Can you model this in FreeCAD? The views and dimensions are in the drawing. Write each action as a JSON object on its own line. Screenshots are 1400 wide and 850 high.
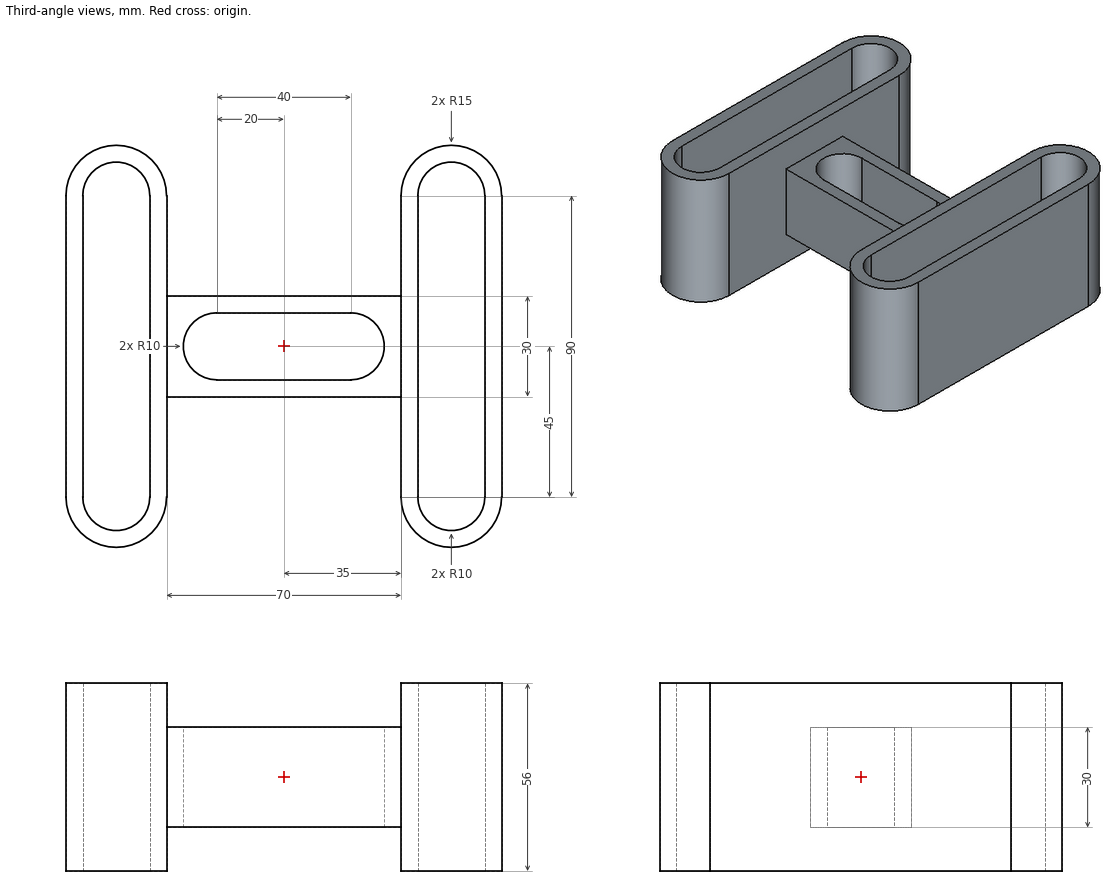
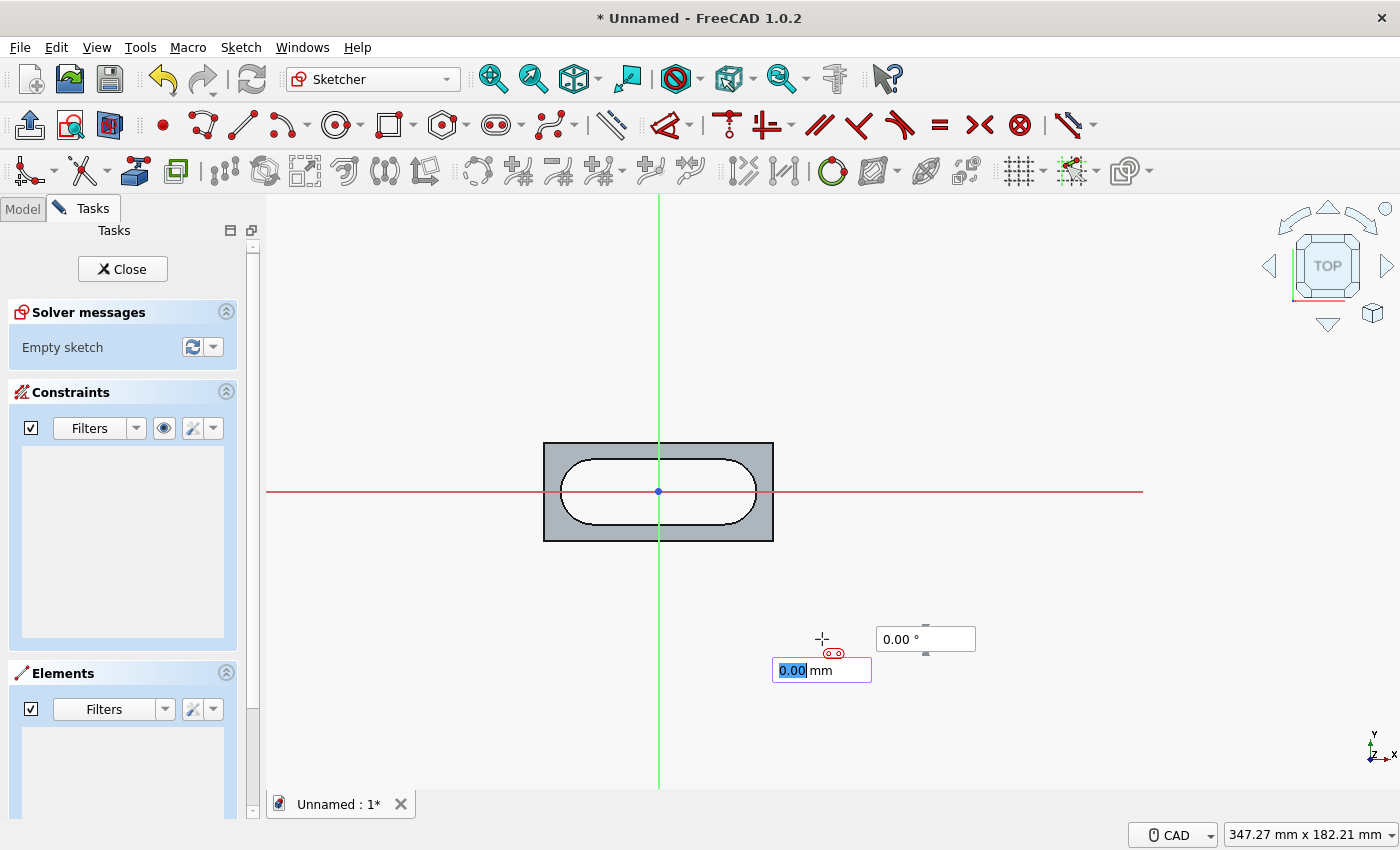
{"action": "left_click", "coordinate": [822, 345]}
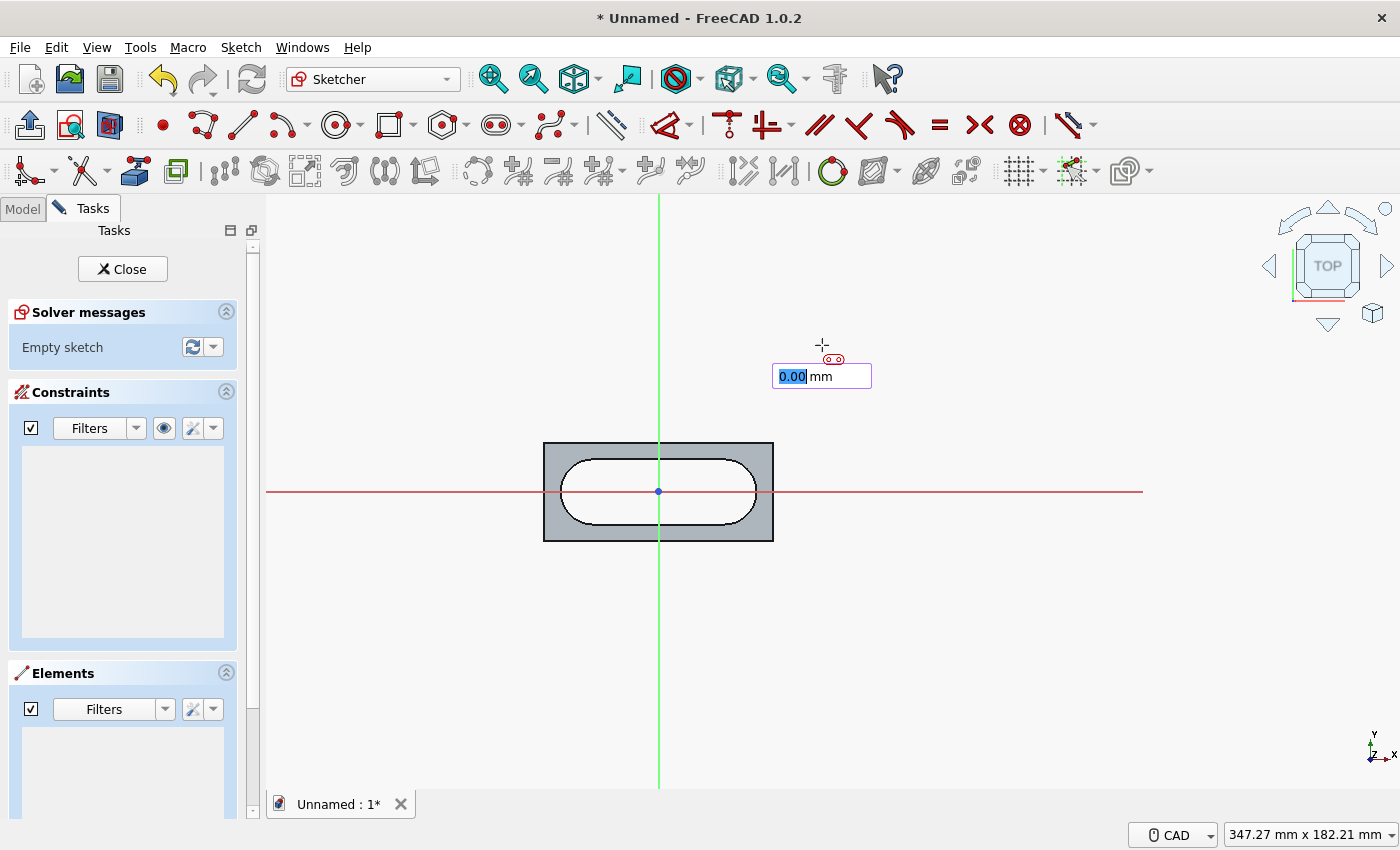
{"action": "left_click", "coordinate": [773, 448]}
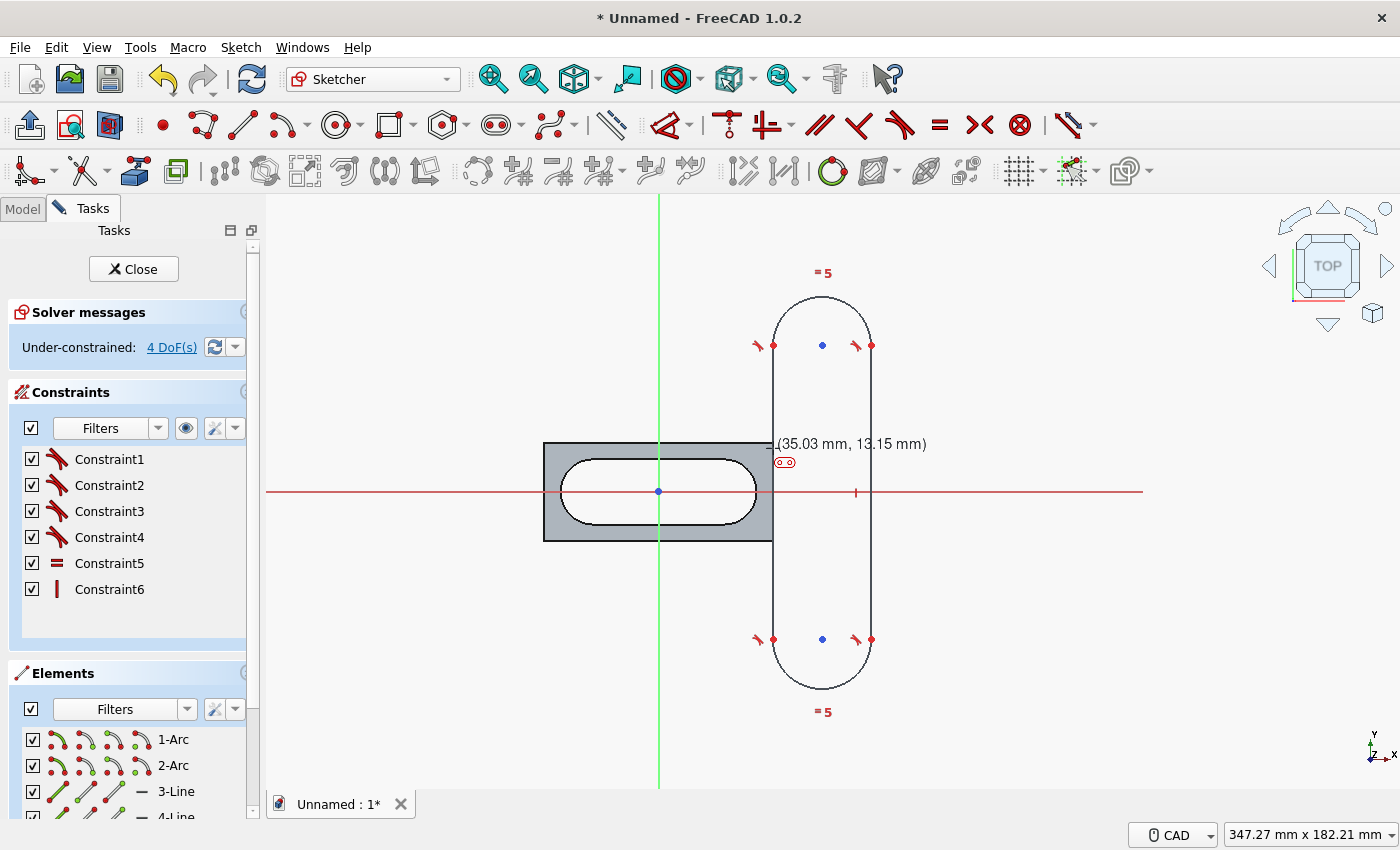
{"action": "left_click", "coordinate": [822, 640]}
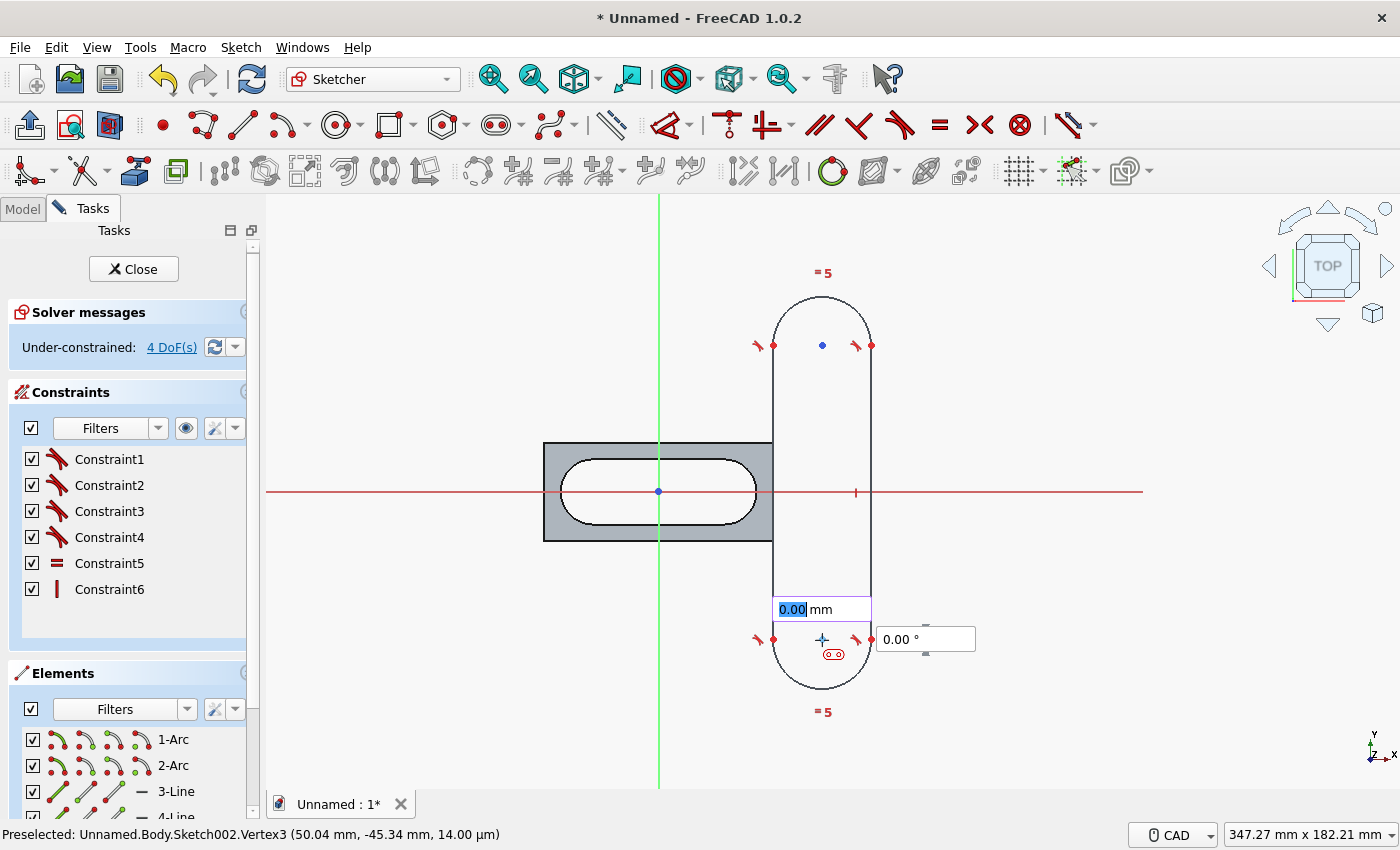
{"action": "left_click", "coordinate": [822, 346]}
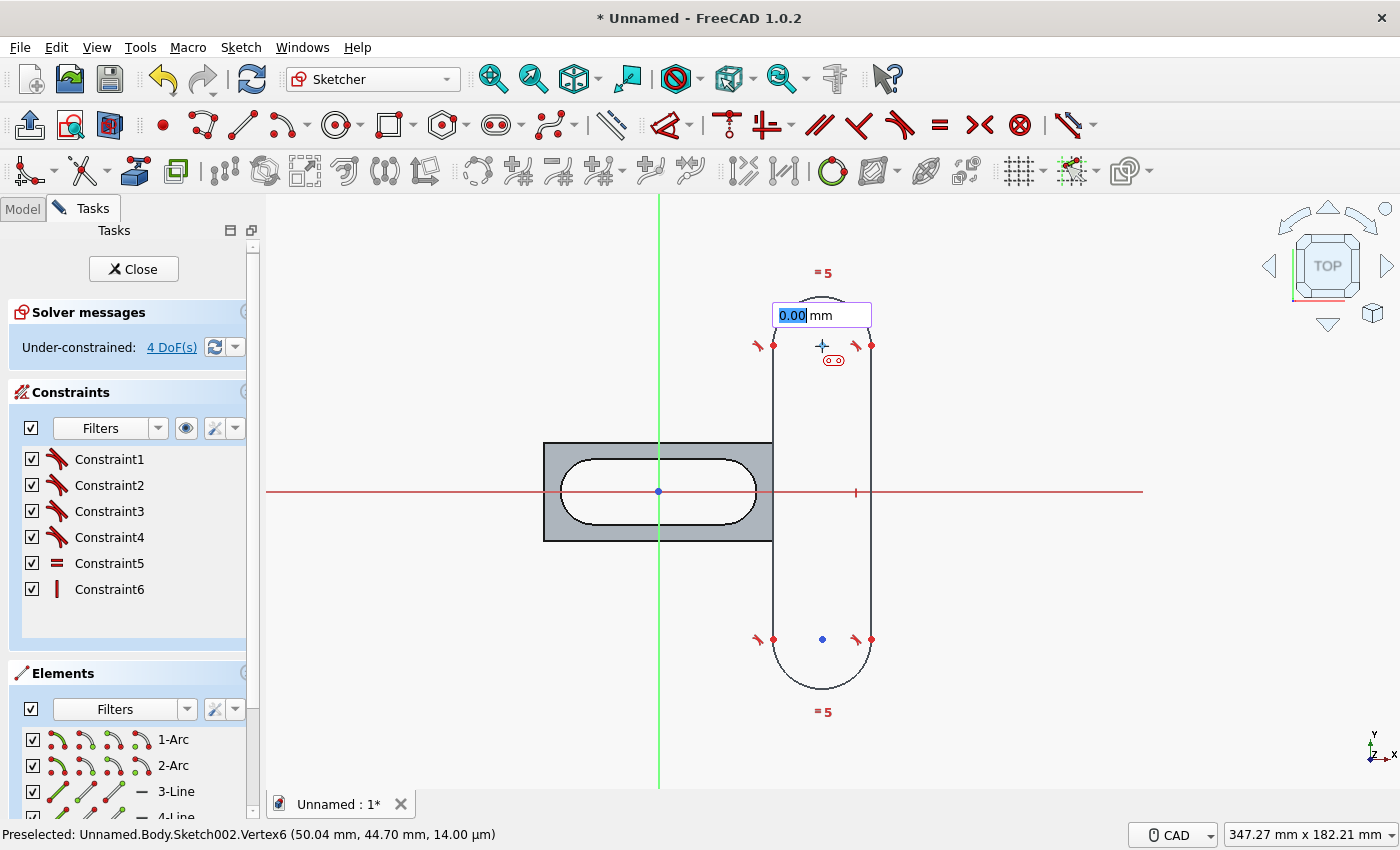
{"action": "left_click", "coordinate": [855, 448]}
{"action": "key", "text": "Escape"}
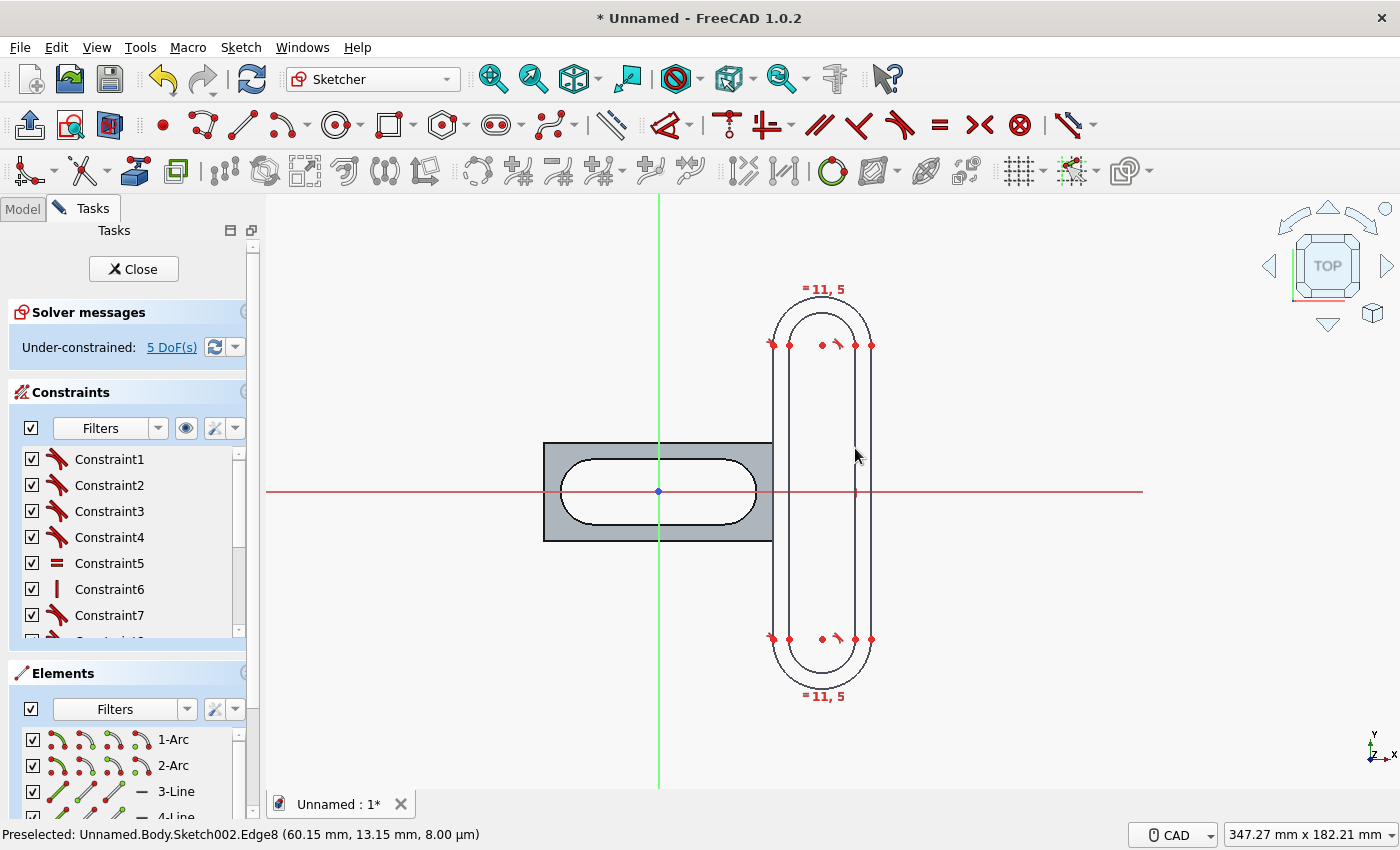
{"action": "left_click", "coordinate": [793, 680]}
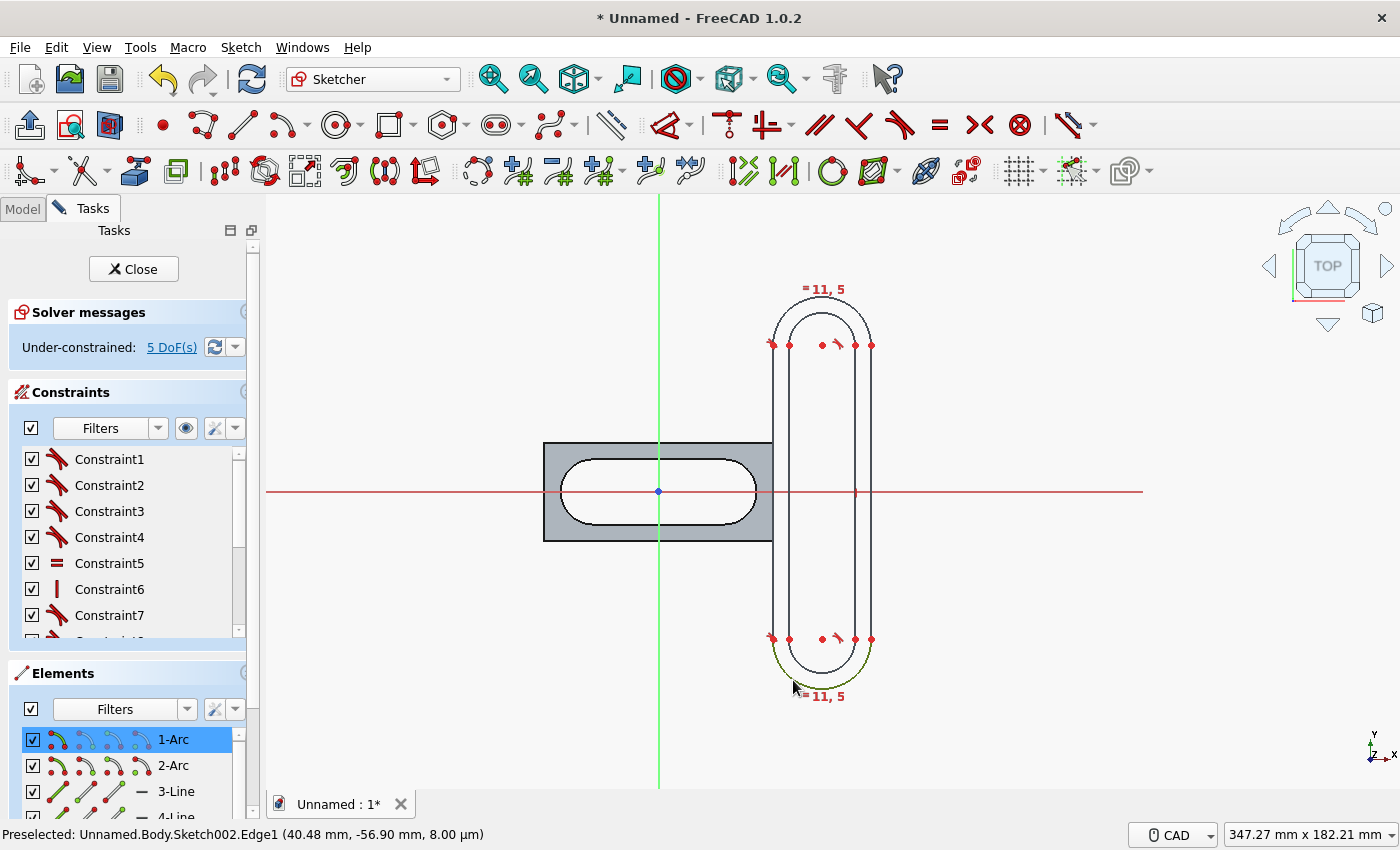
{"action": "key", "text": "k r"}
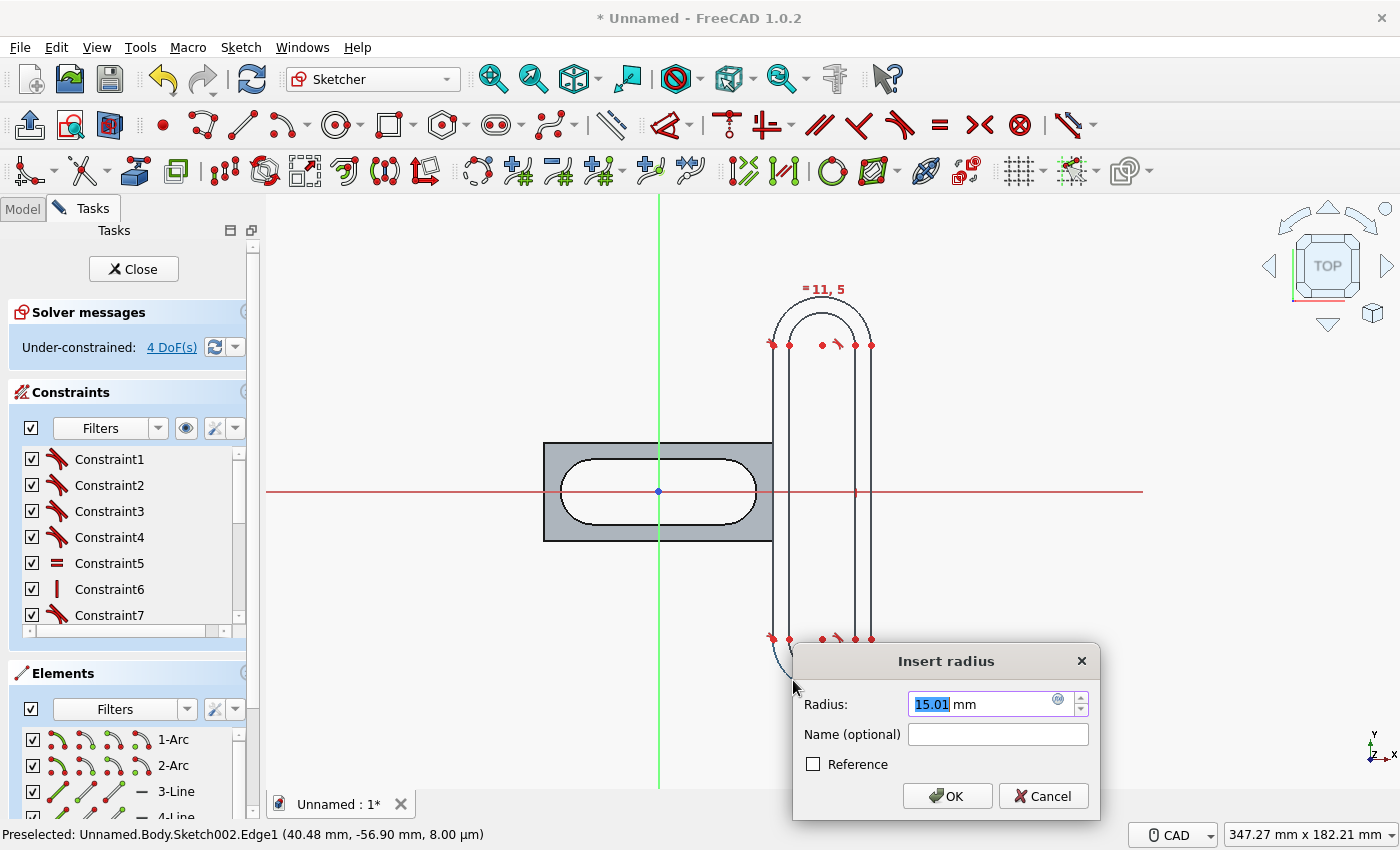
{"action": "type", "text": "15"}
{"action": "key", "text": "Return"}